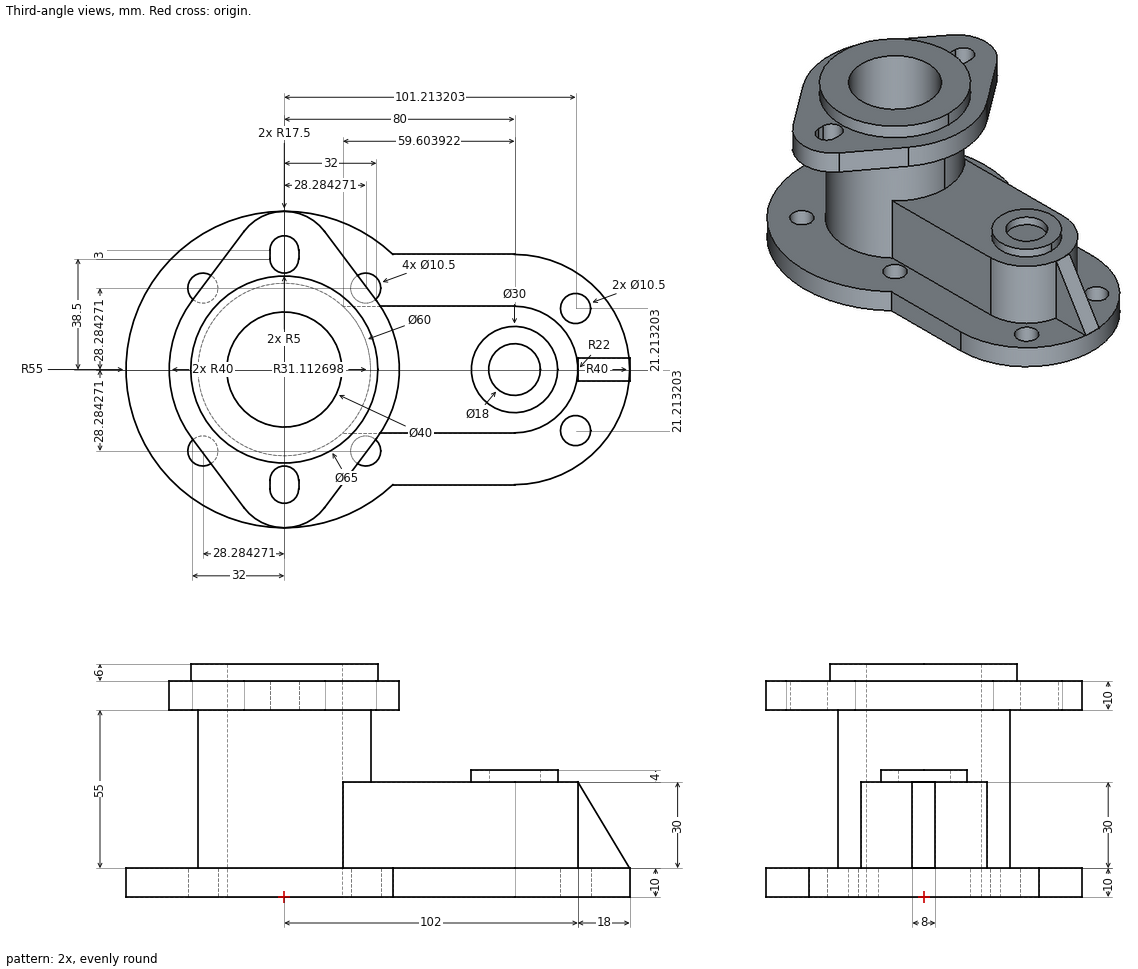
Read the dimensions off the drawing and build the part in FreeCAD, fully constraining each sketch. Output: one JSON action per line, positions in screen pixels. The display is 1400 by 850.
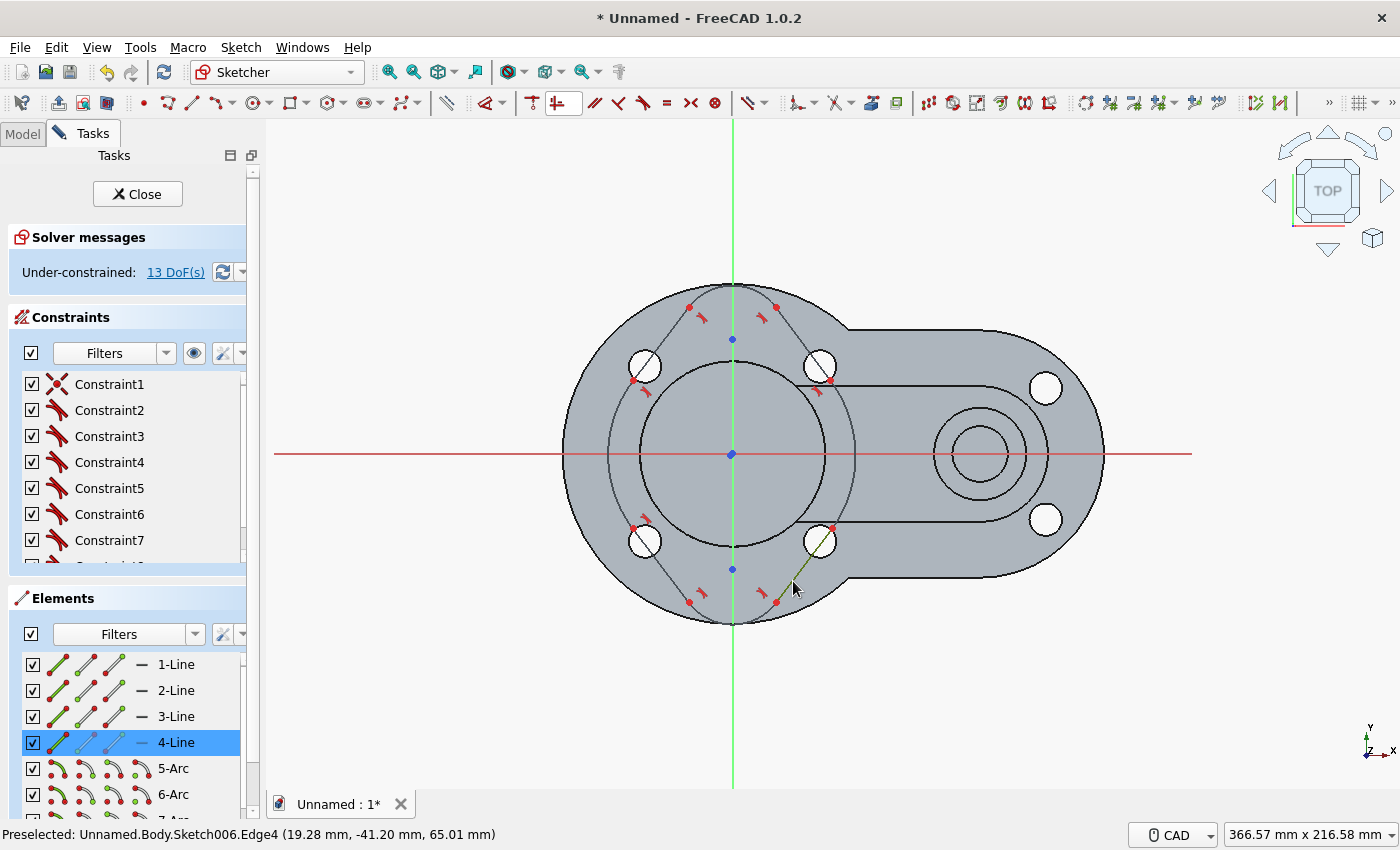
{"action": "left_click", "coordinate": [852, 486]}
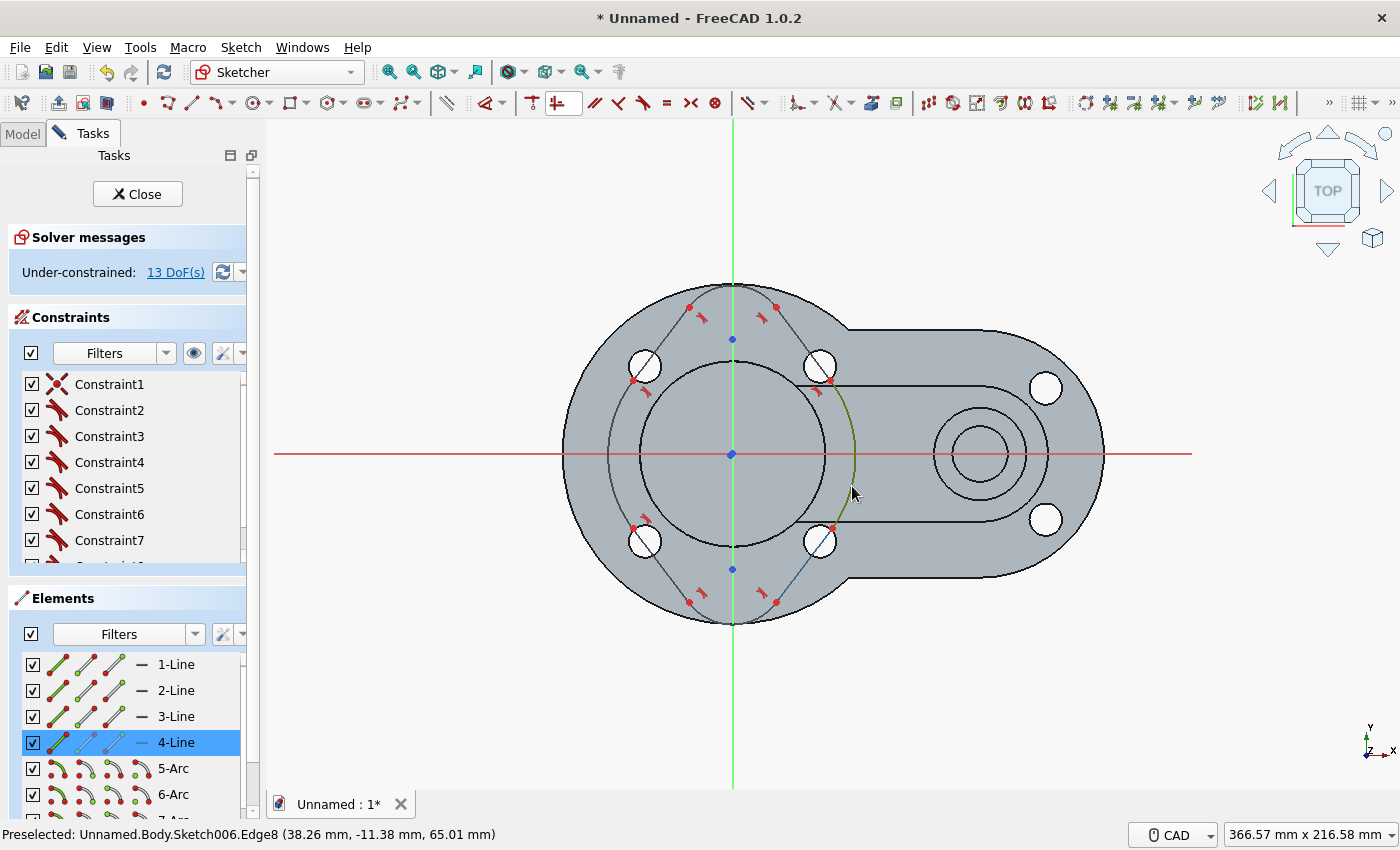
{"action": "left_click", "coordinate": [644, 104]}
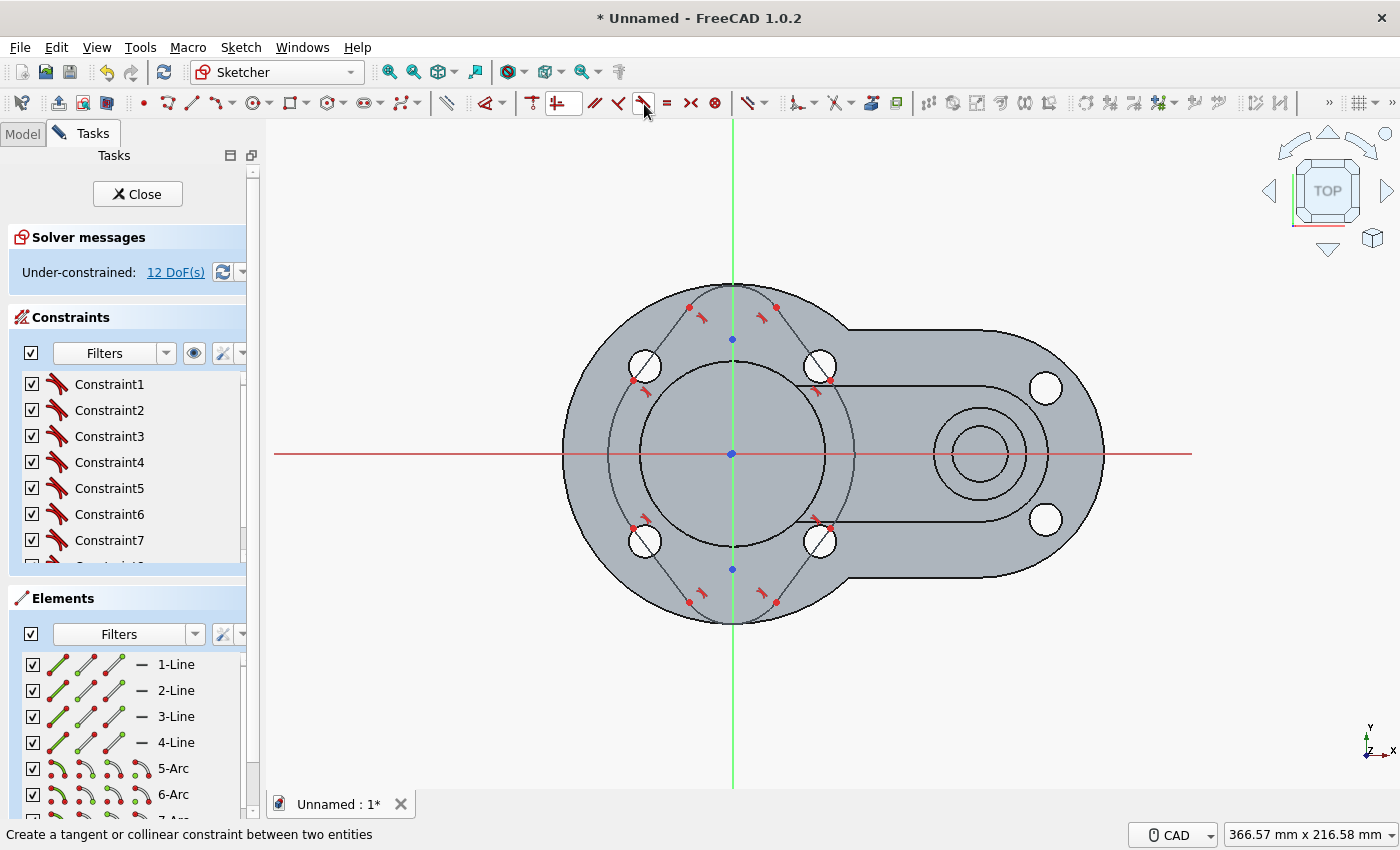
{"action": "left_click", "coordinate": [612, 424]}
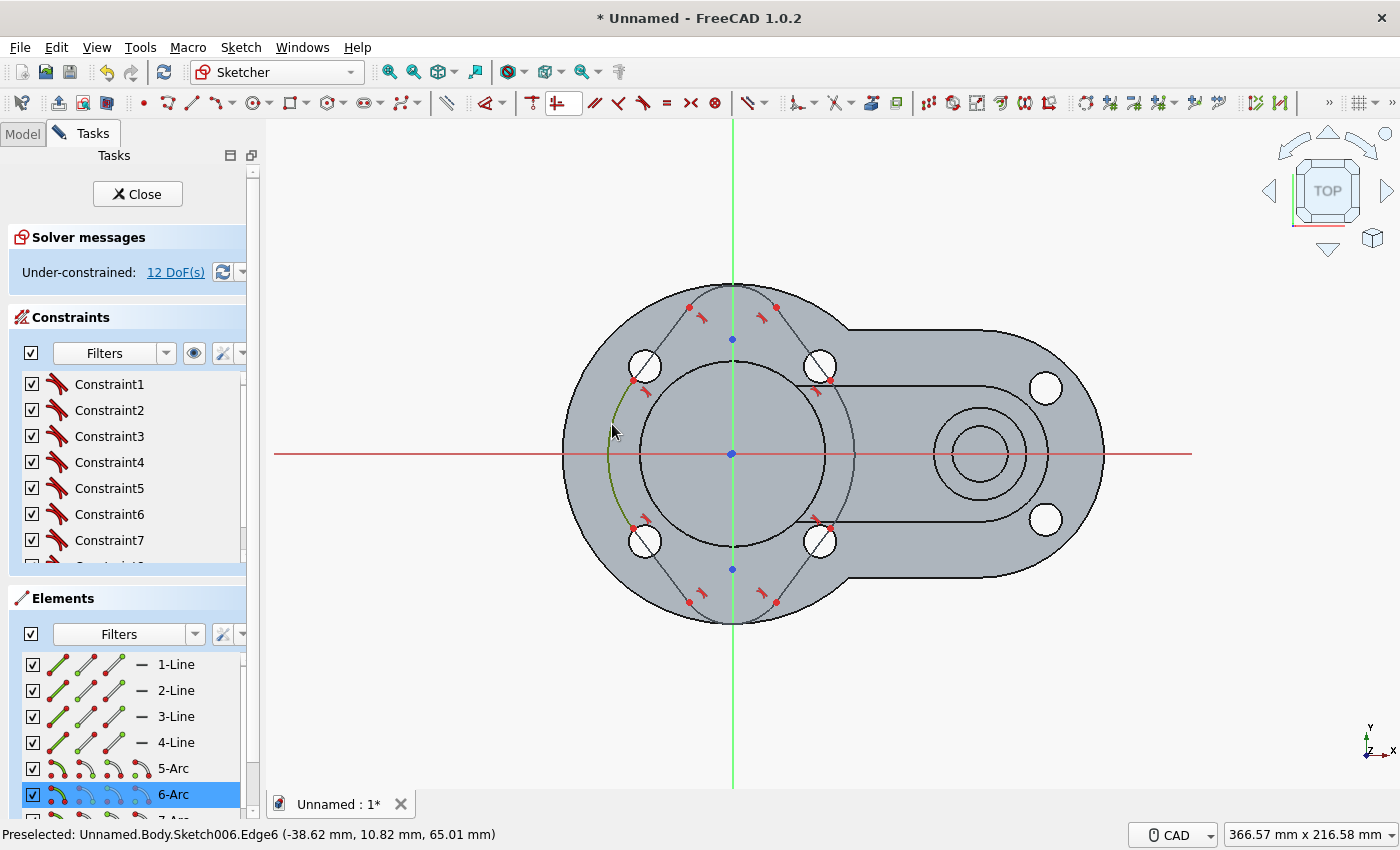
{"action": "left_click", "coordinate": [851, 486]}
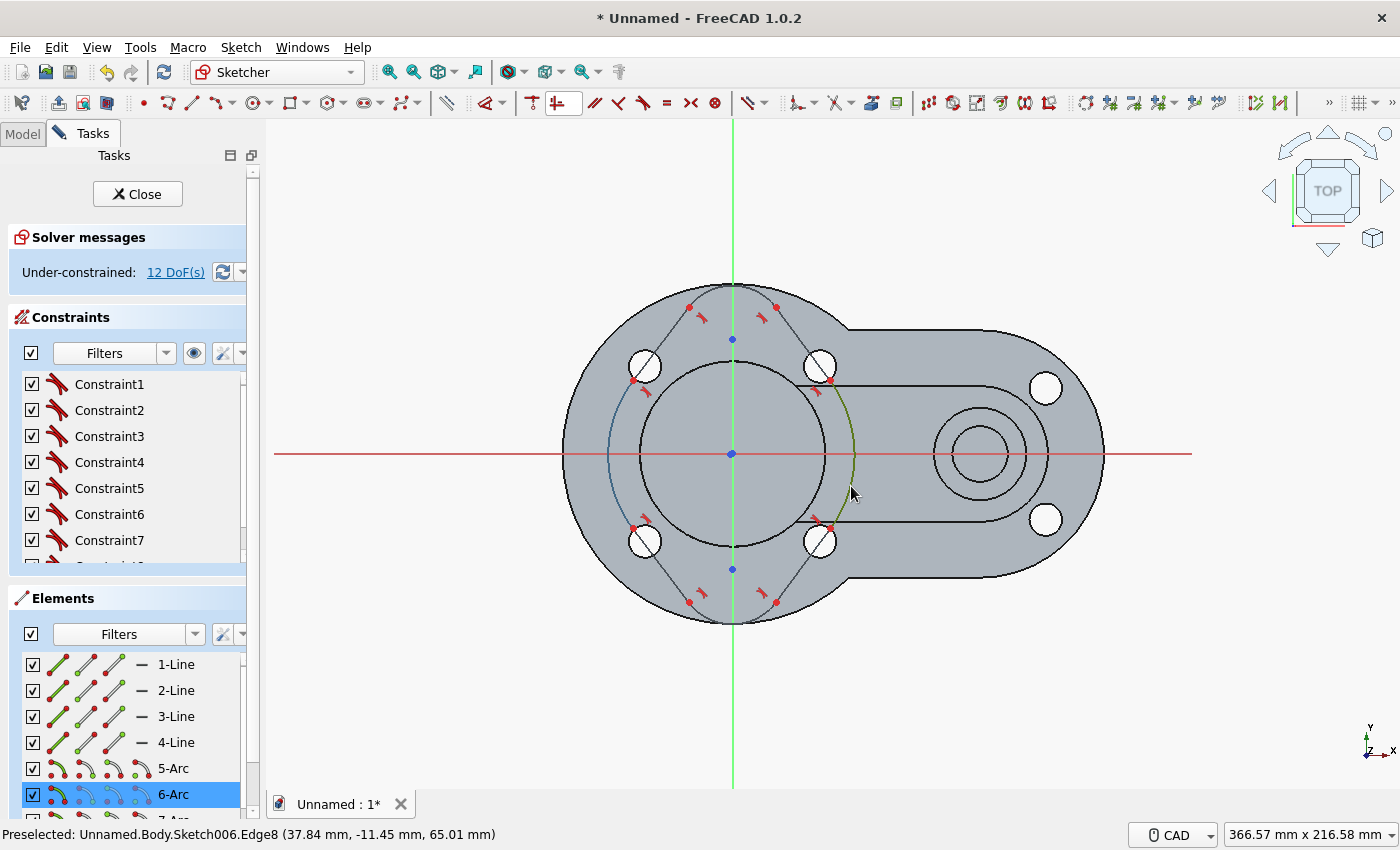
{"action": "key", "text": "c"}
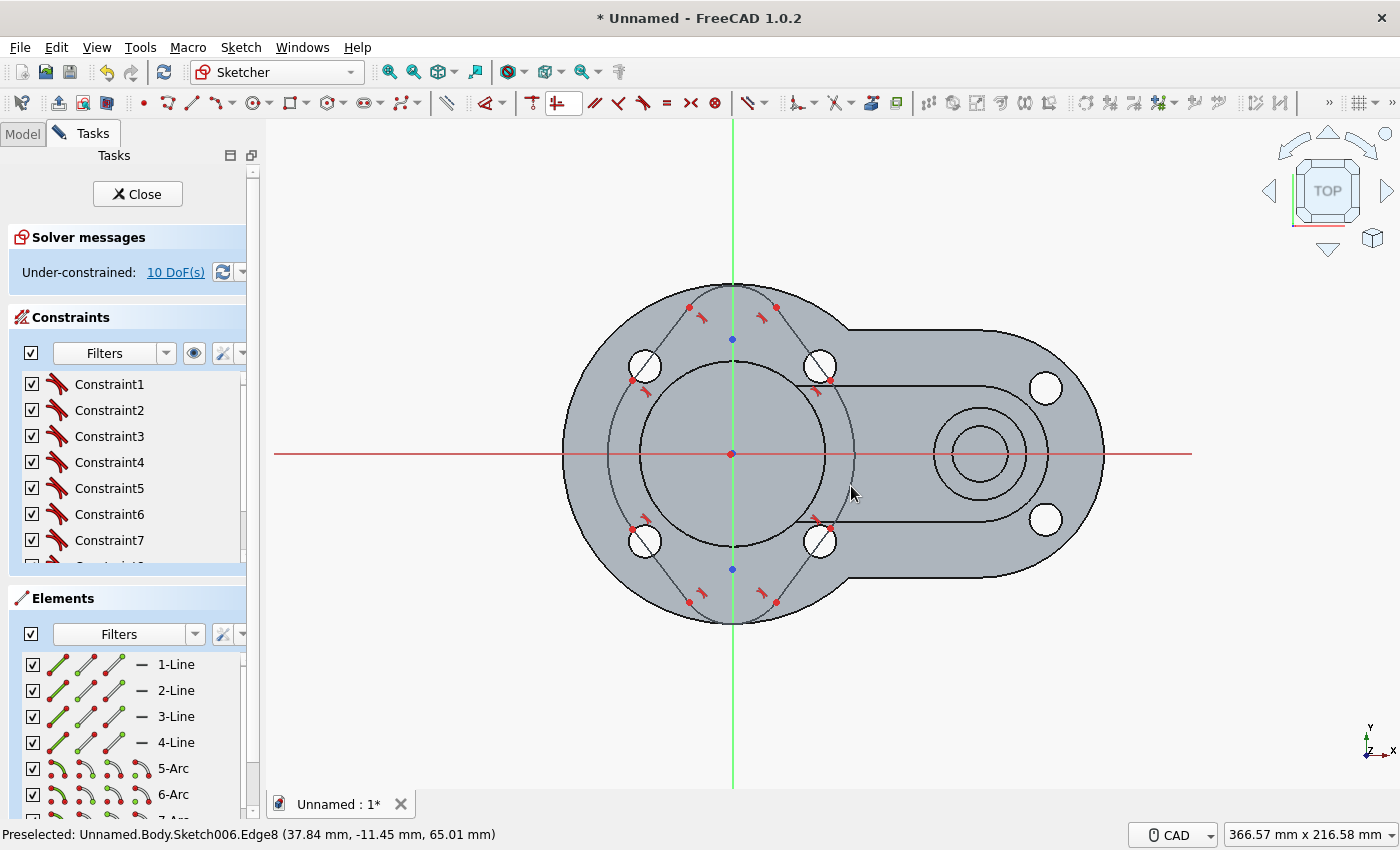
{"action": "left_click_drag", "start_coordinate": [720, 444], "coordinate": [743, 465]}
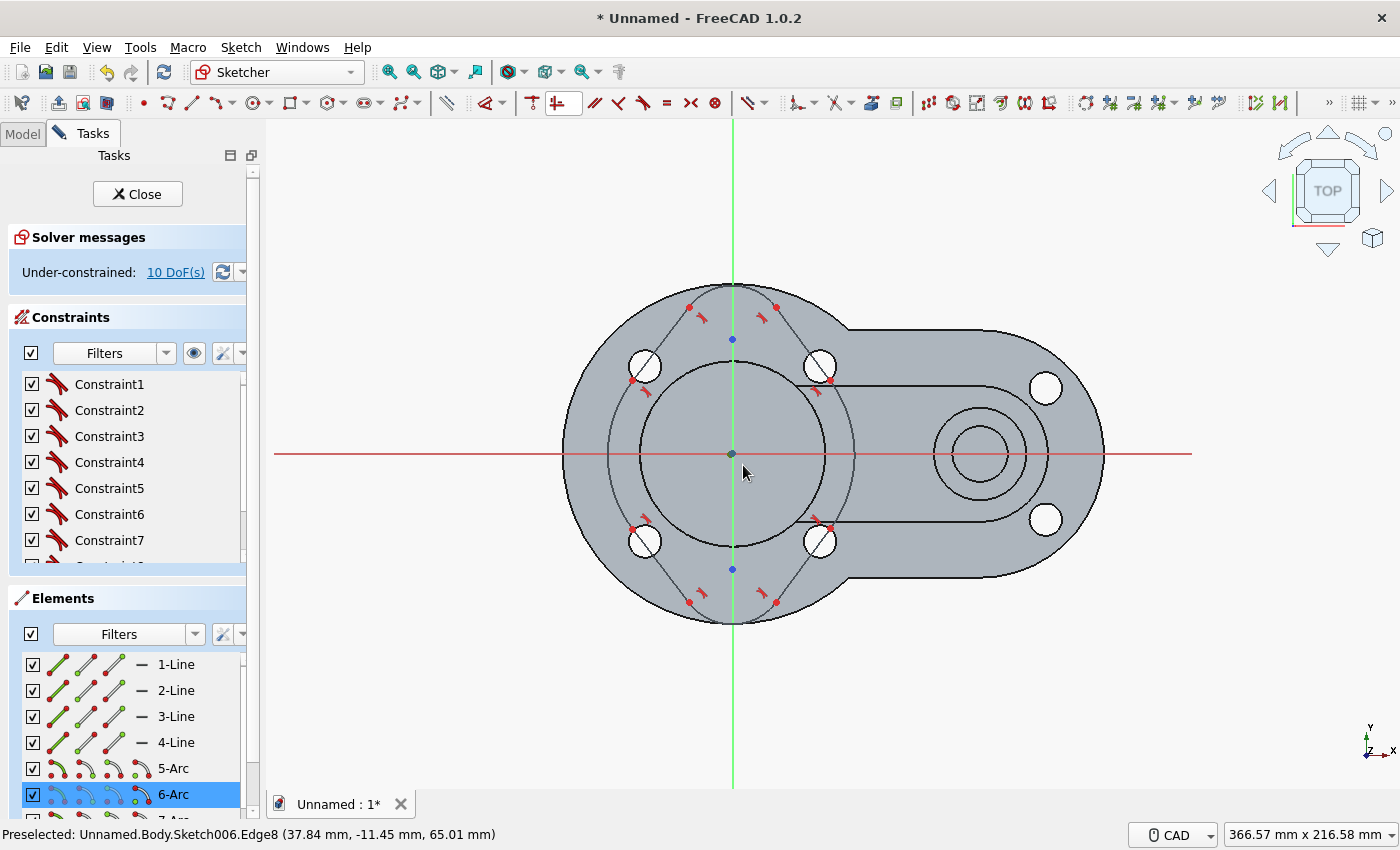
{"action": "key", "text": "c"}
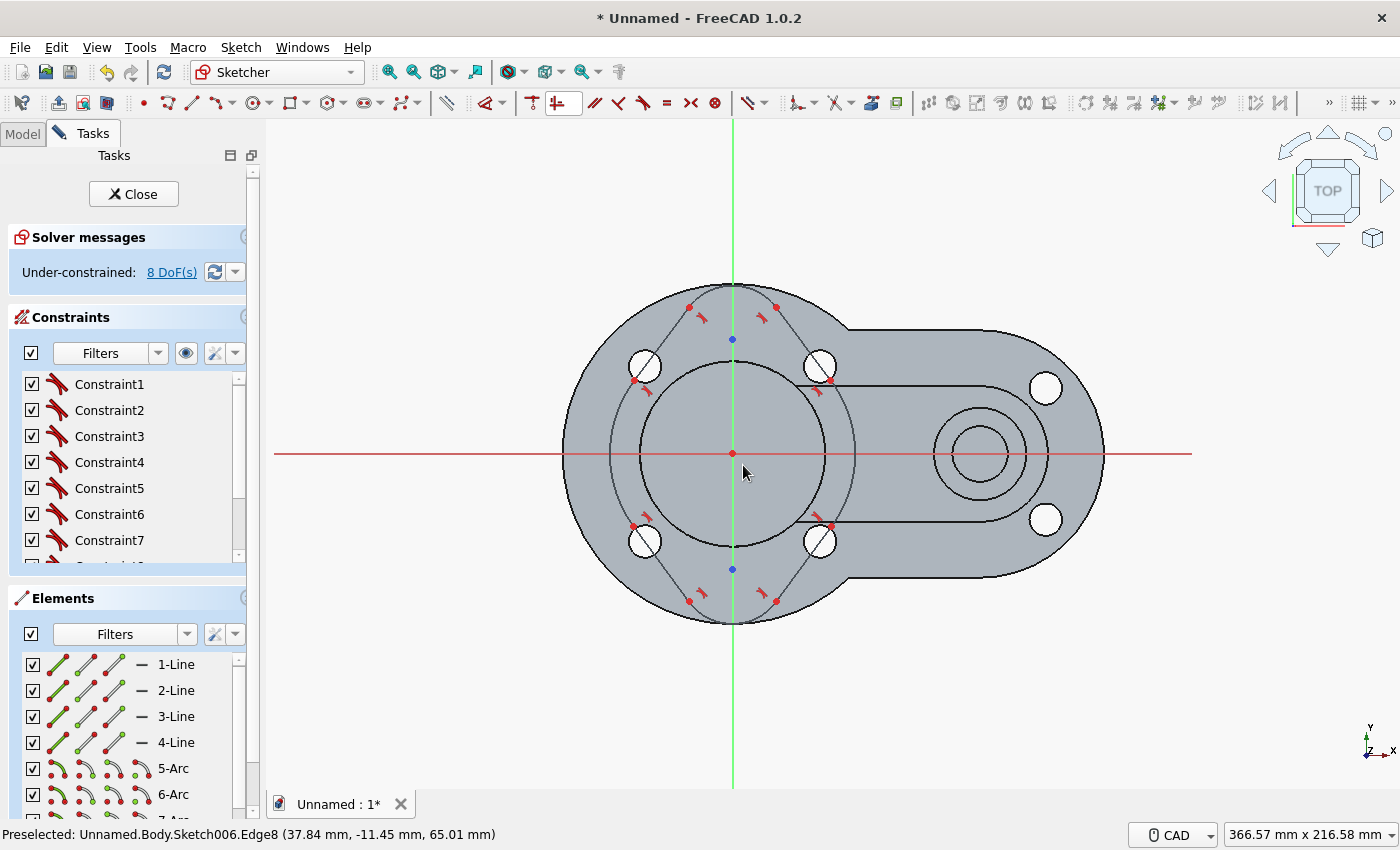
{"action": "left_click", "coordinate": [752, 289]}